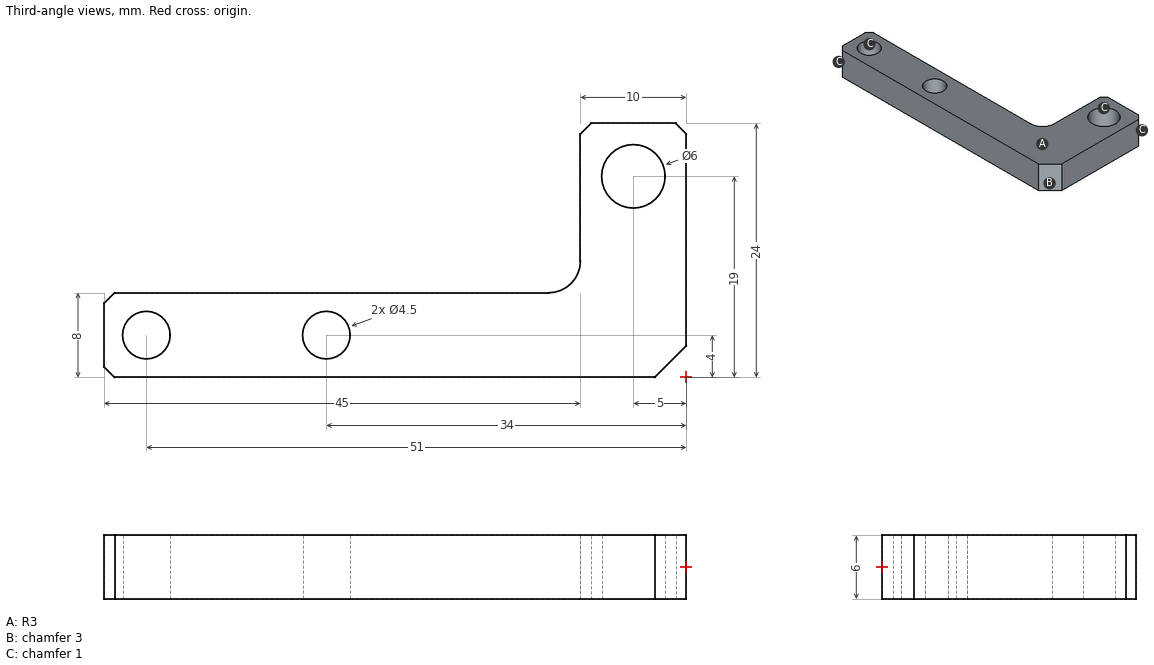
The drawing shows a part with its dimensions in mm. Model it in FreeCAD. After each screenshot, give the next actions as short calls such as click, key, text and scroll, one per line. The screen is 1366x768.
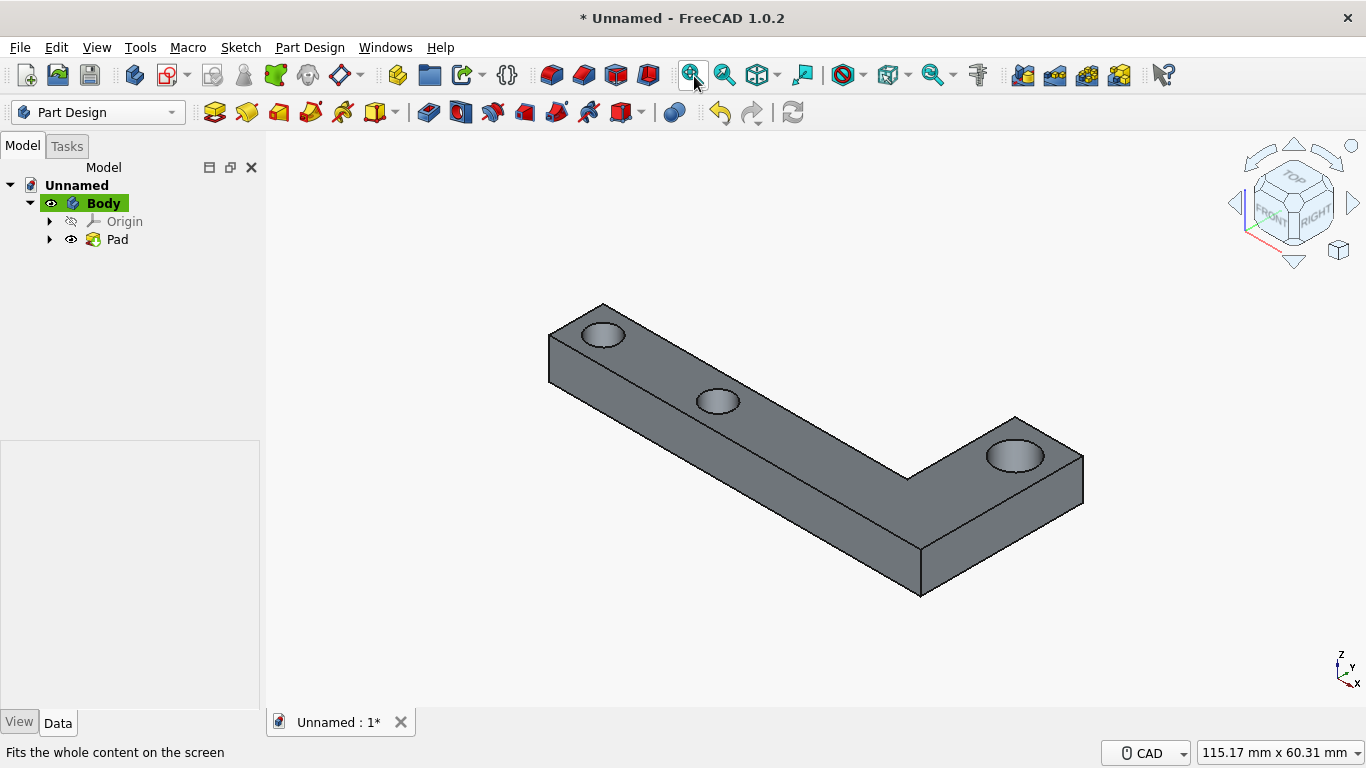
key(2)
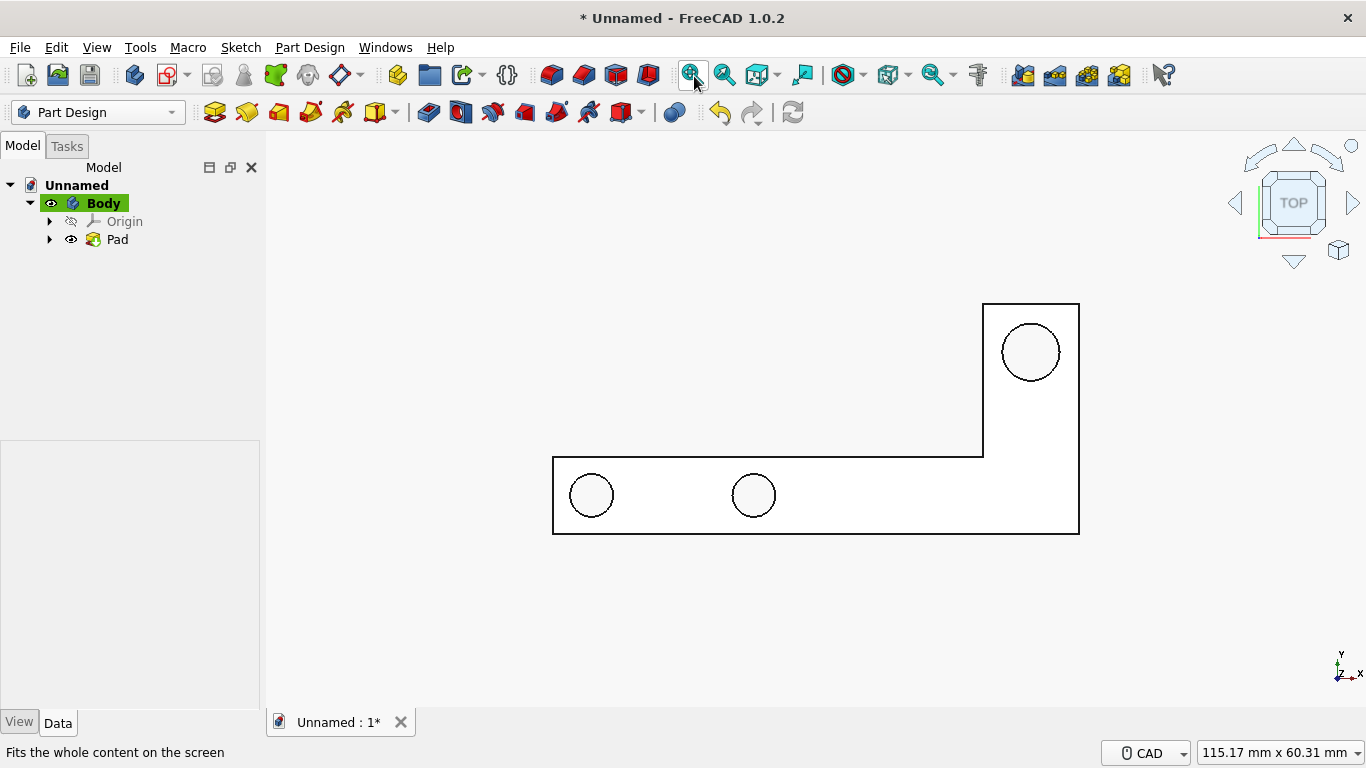
key(1)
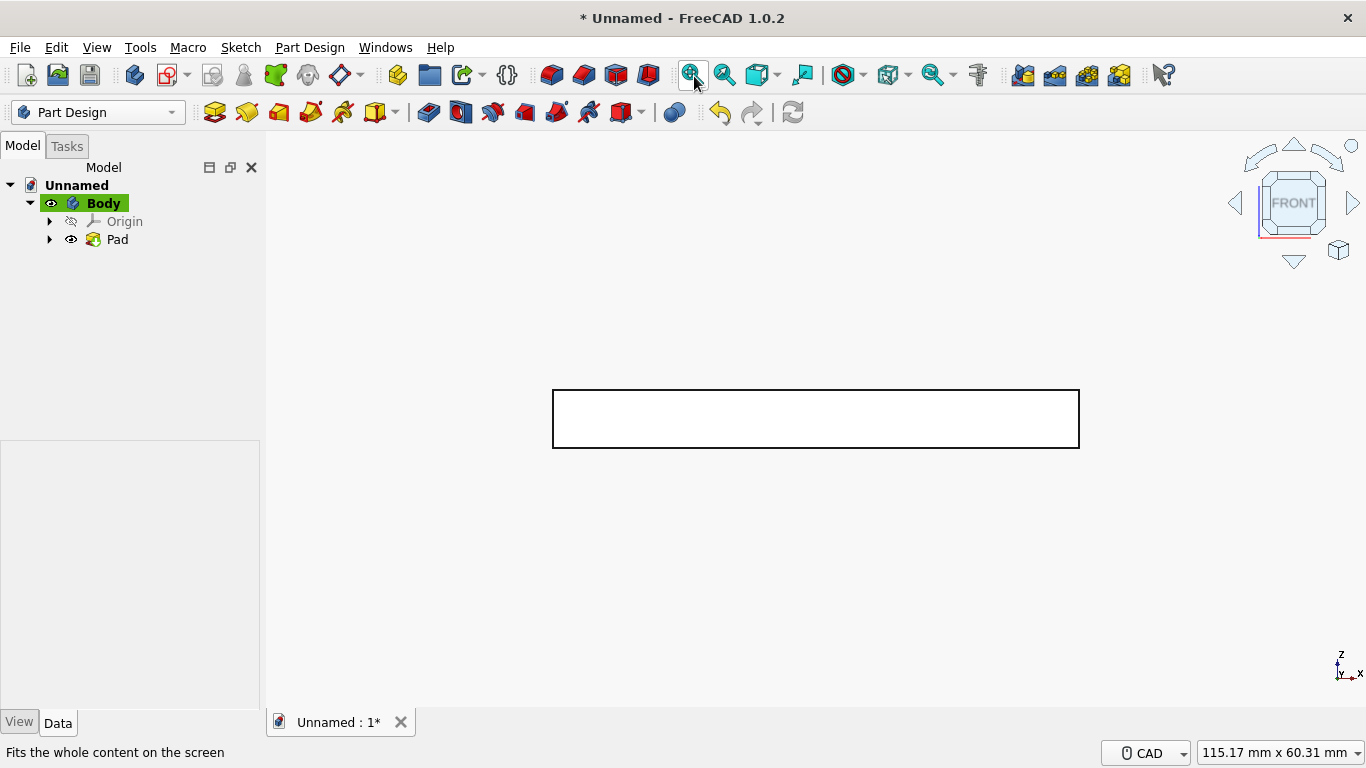
key(3)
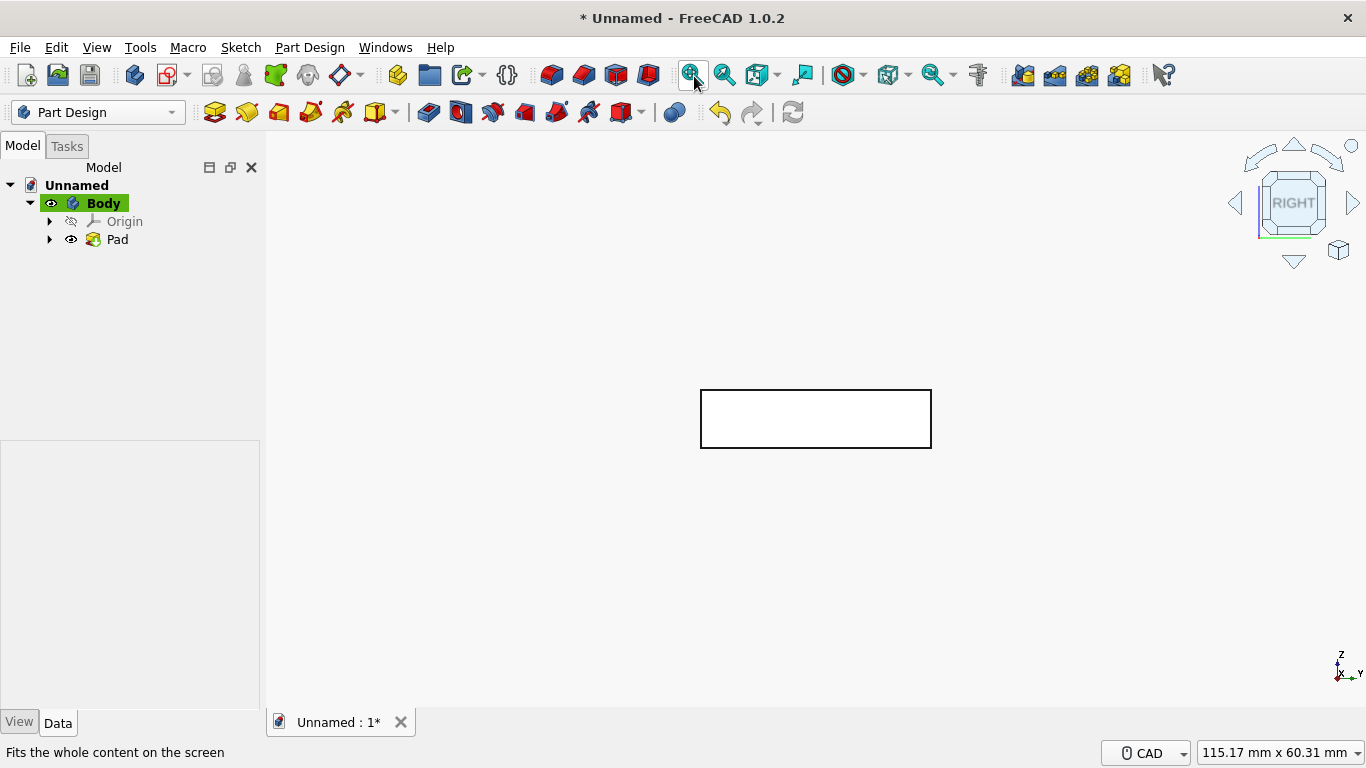
key(v)
key(f)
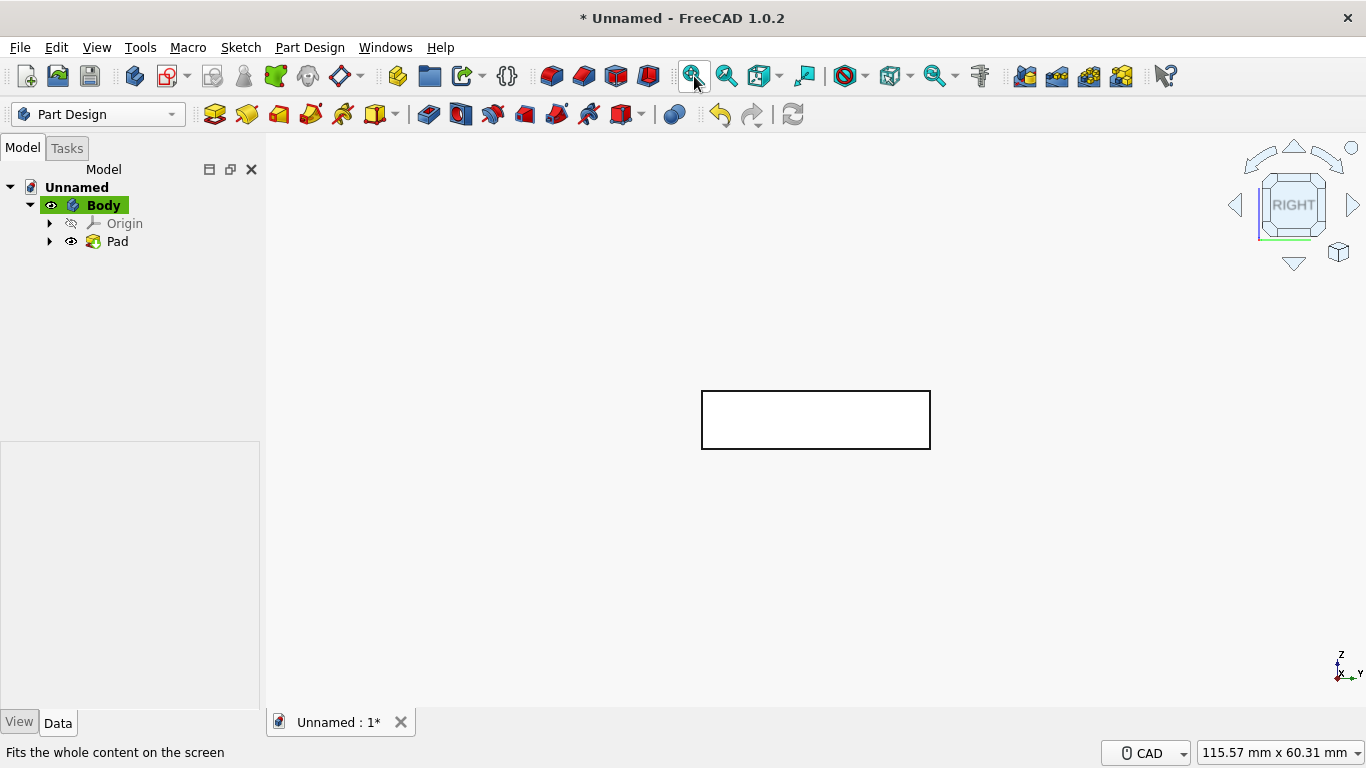
key(5)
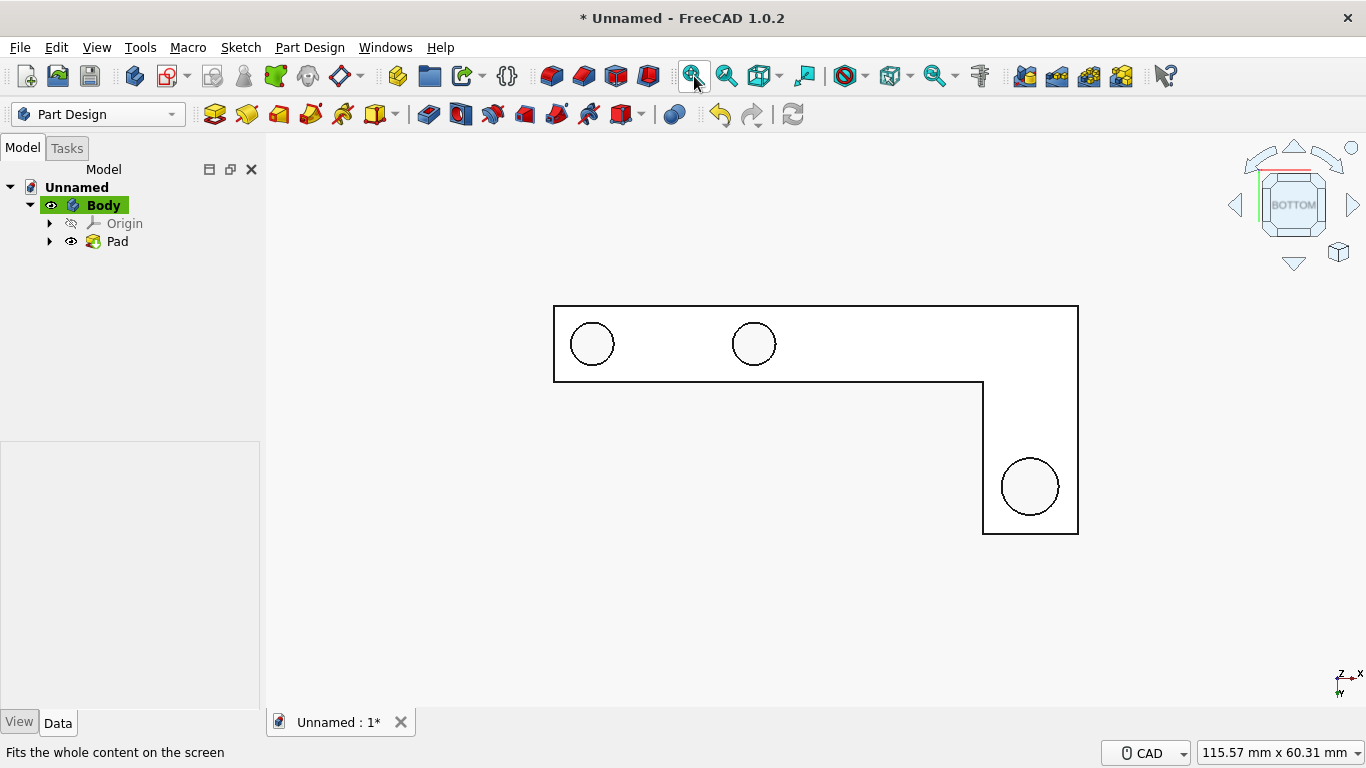
key(4)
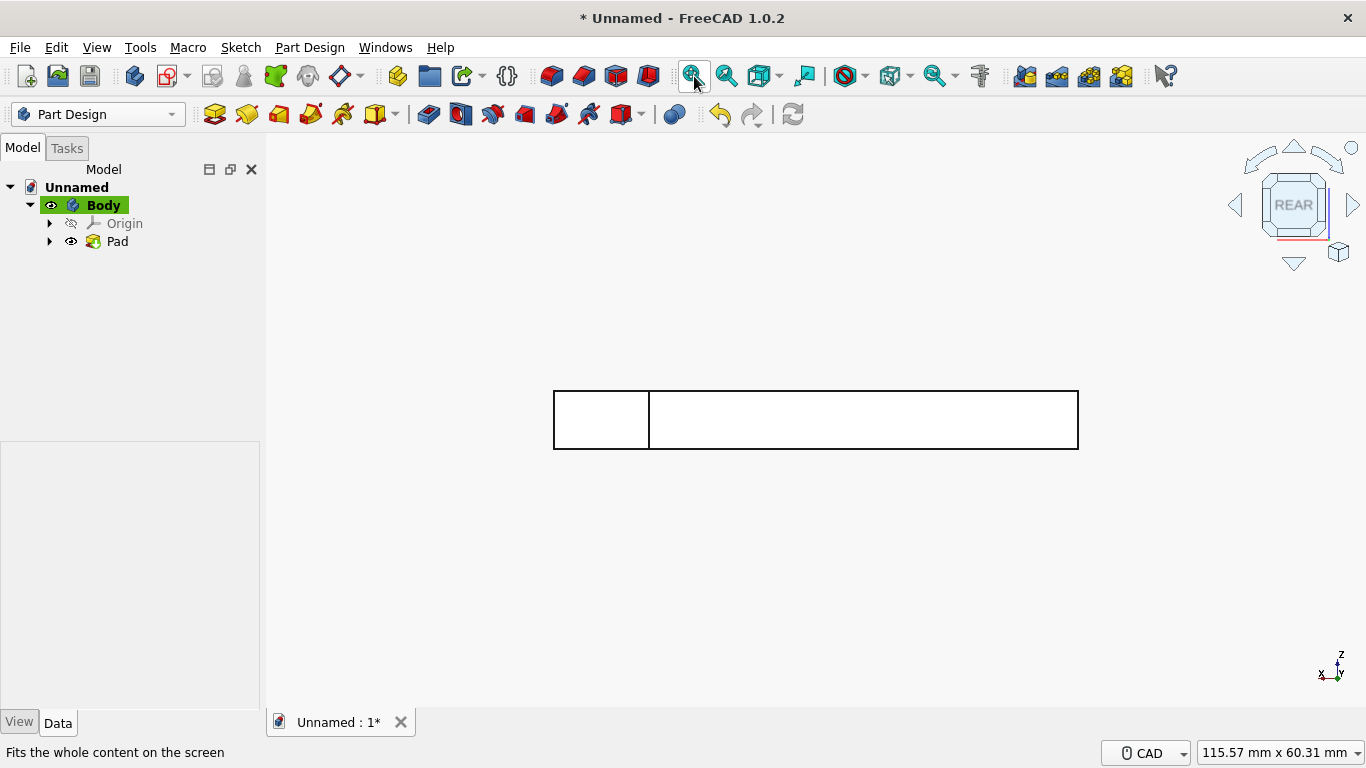
key(6)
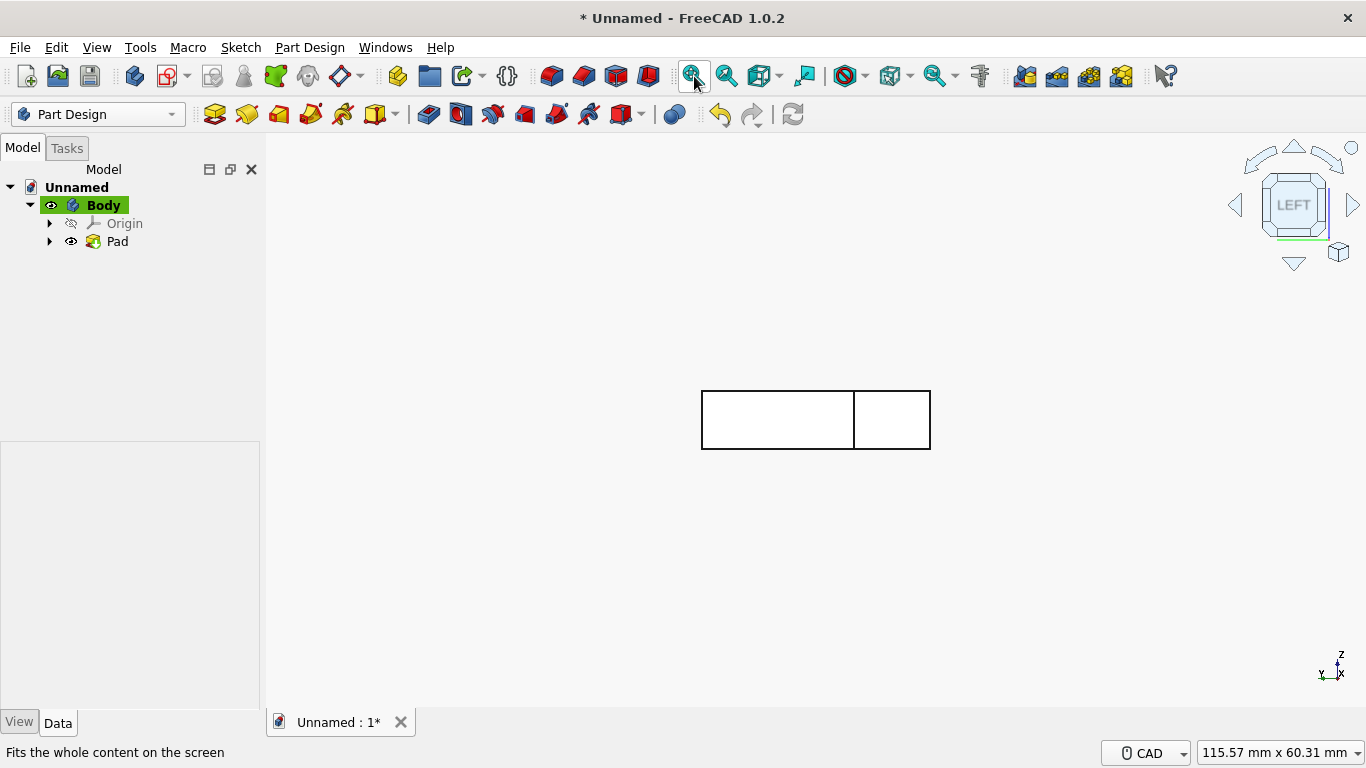
key(v)
key(f)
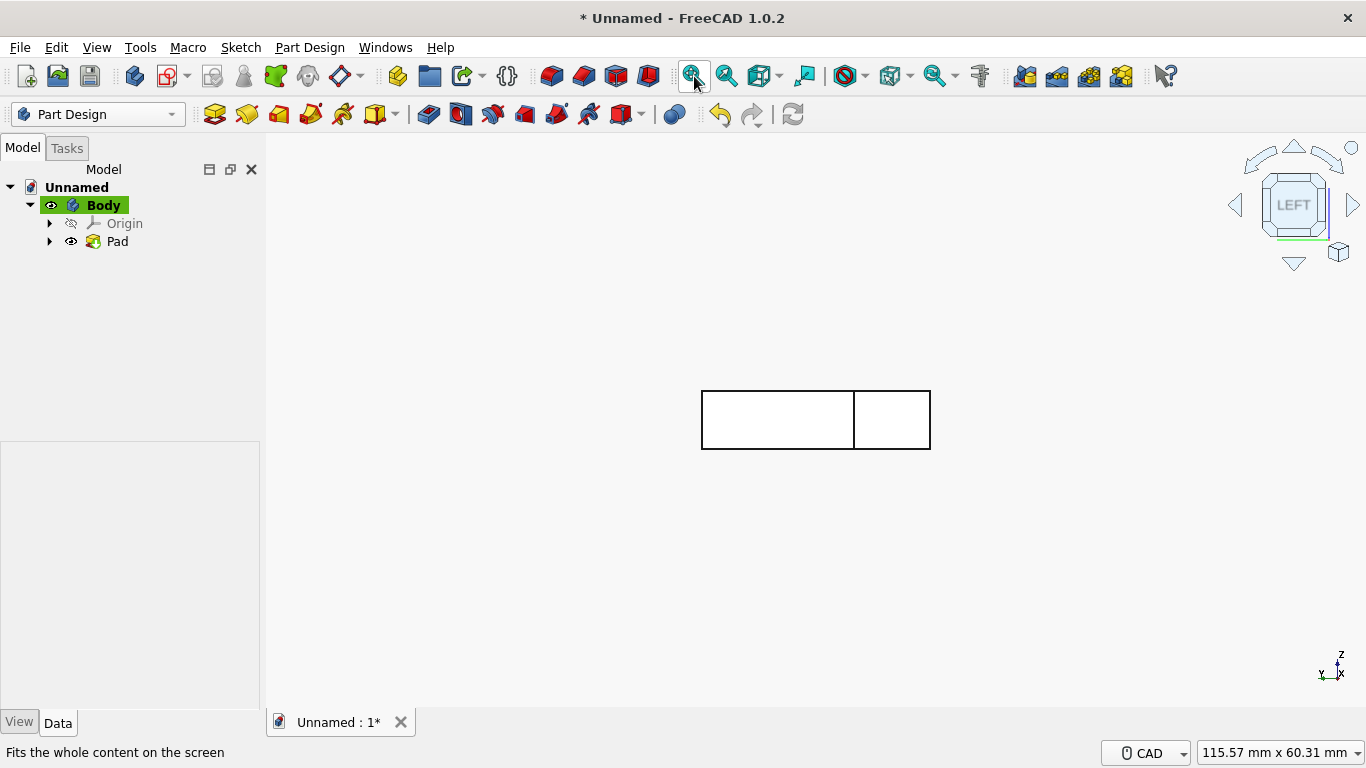
key(v)
key(3)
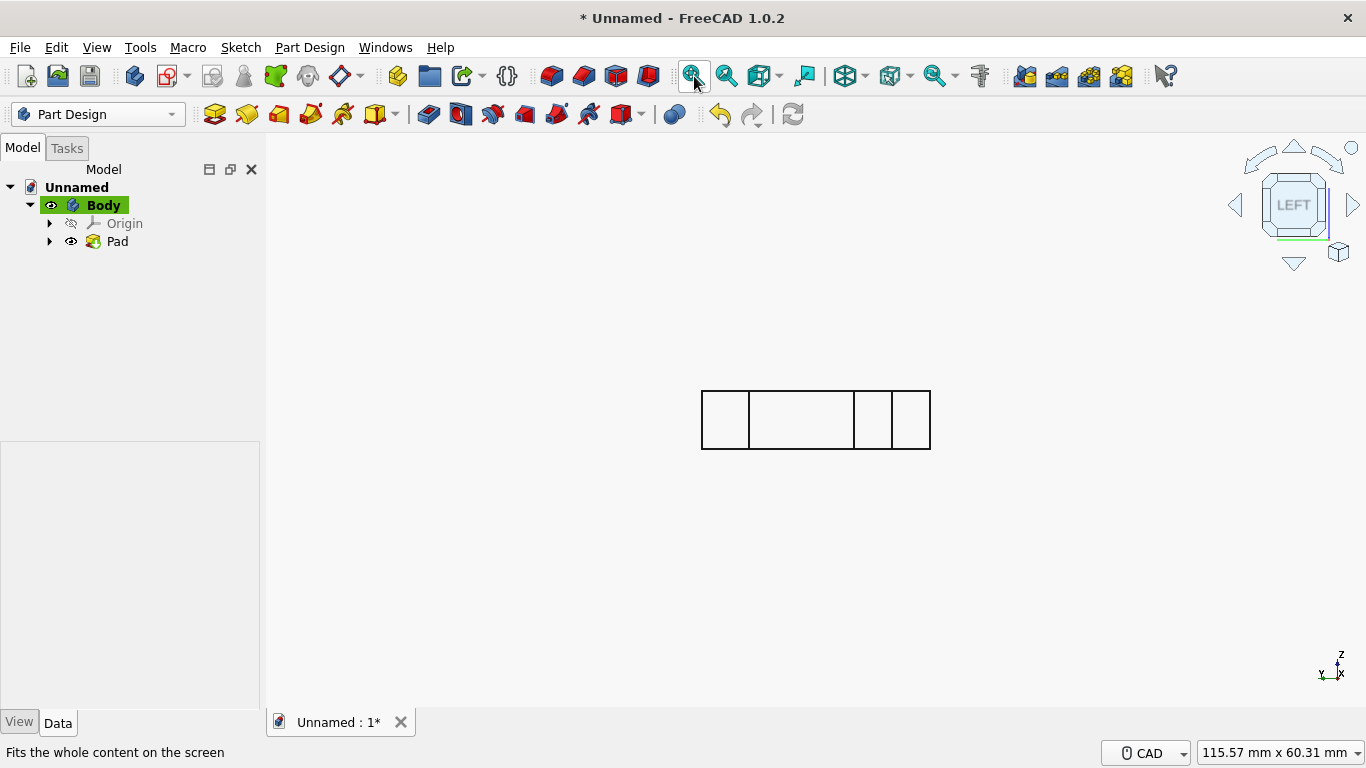
key(0)